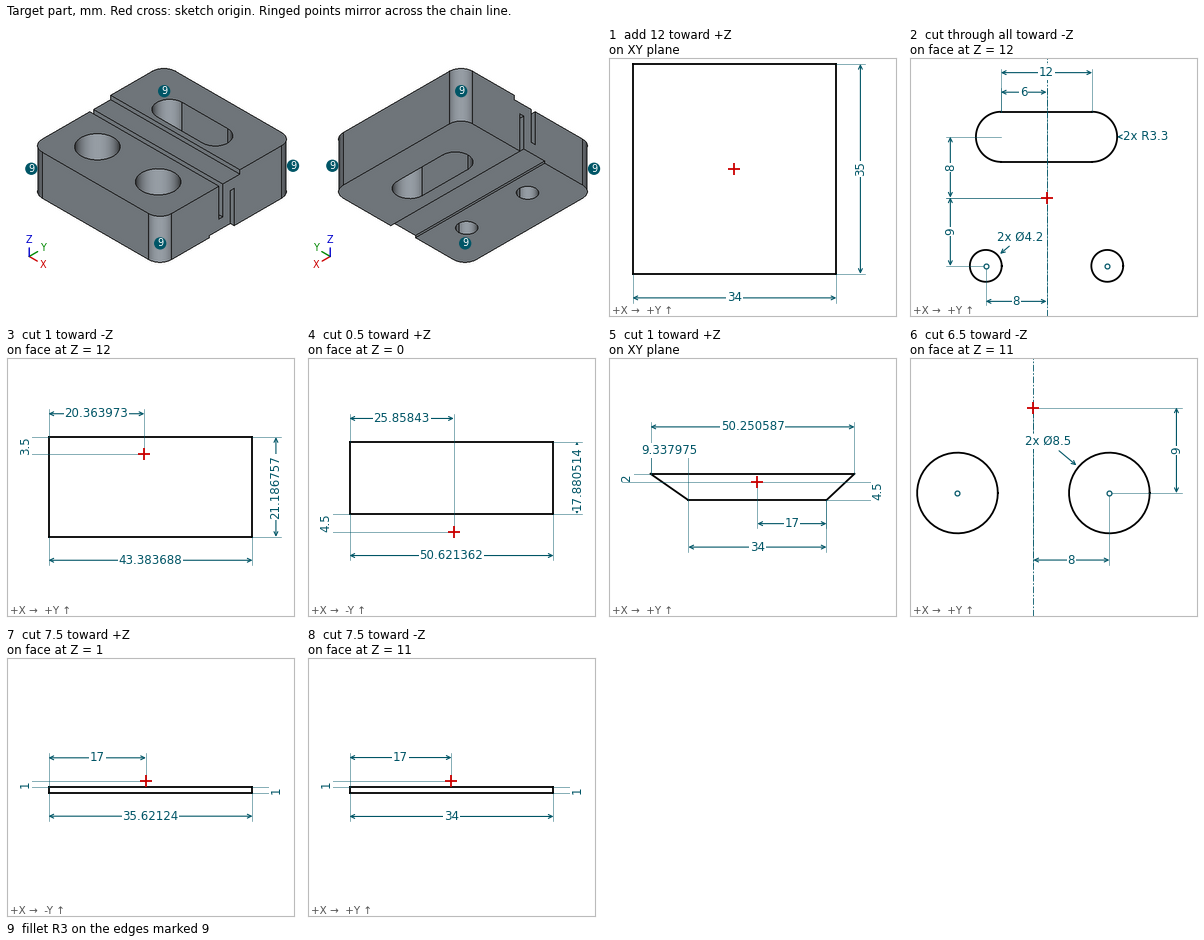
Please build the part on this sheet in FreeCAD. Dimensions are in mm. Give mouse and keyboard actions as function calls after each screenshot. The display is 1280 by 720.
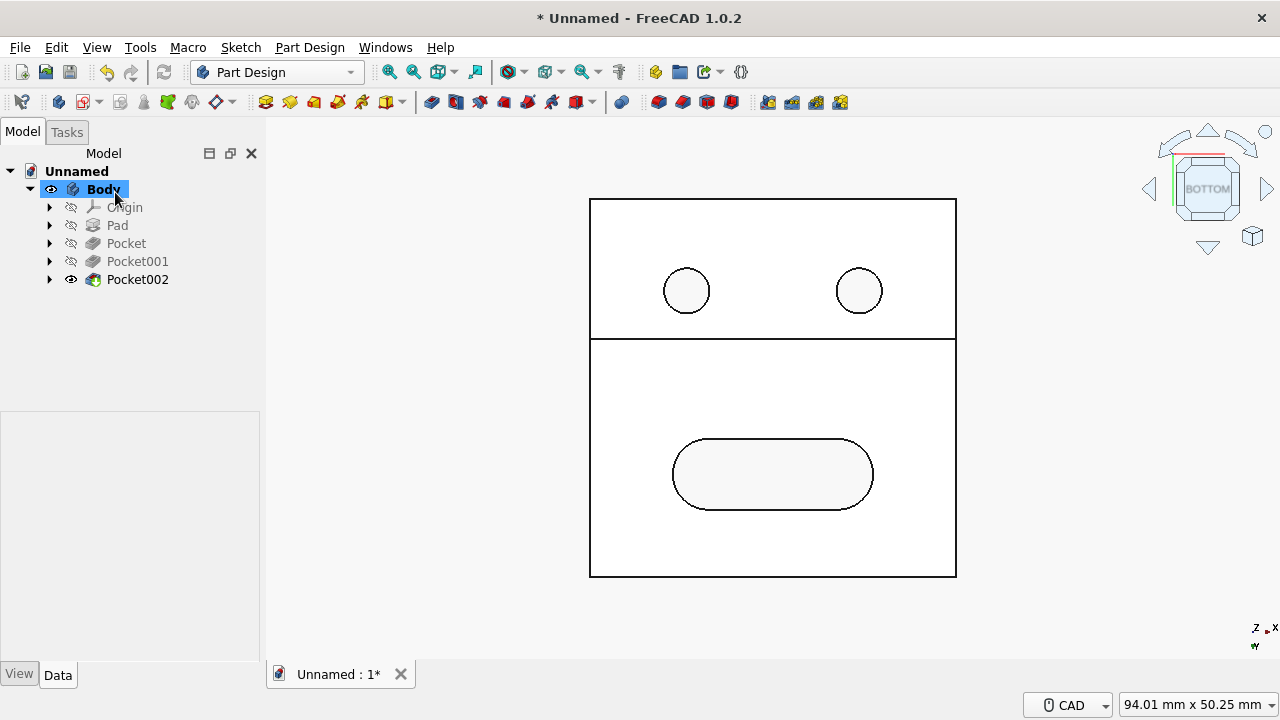
click(84, 102)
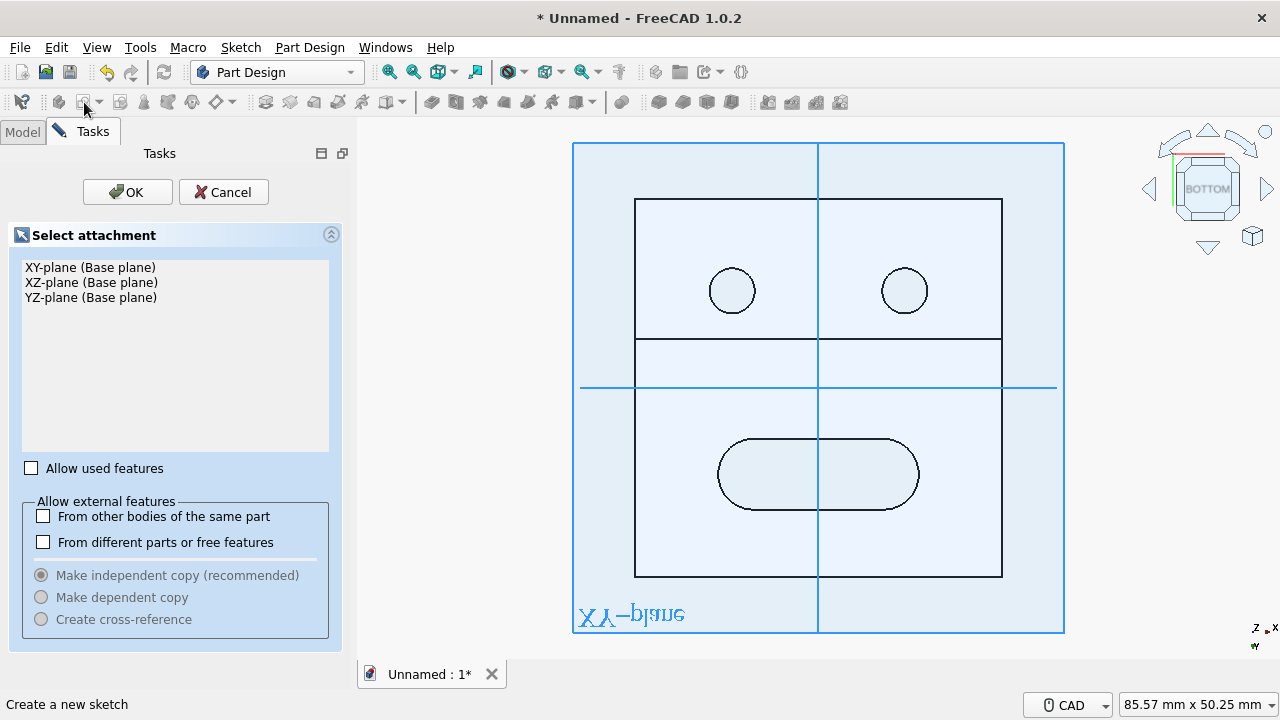
click(82, 268)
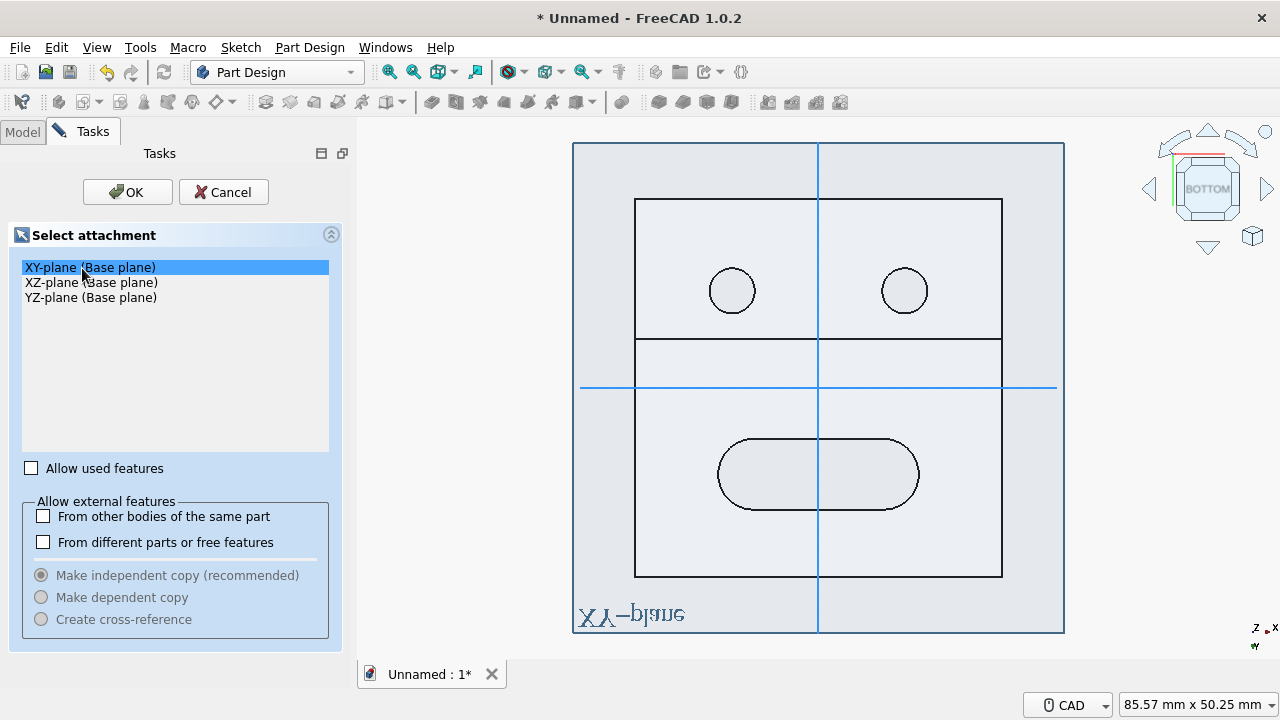
click(128, 192)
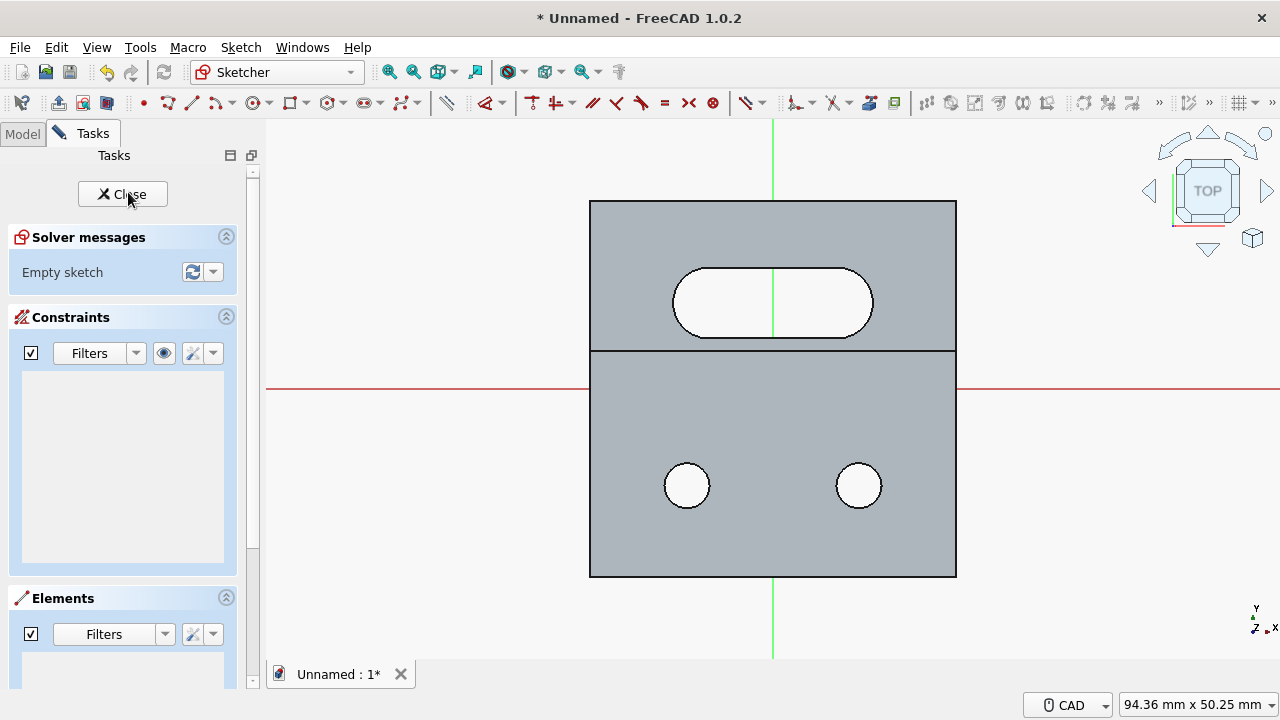
click(108, 104)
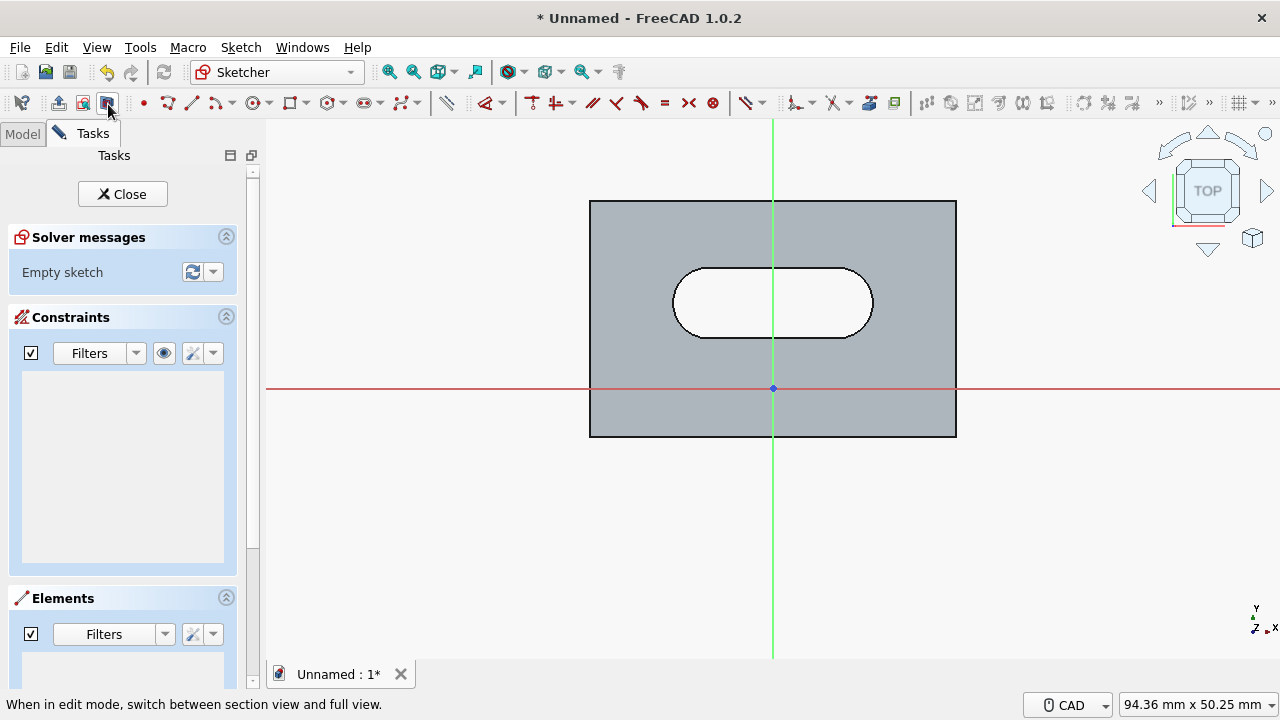
key(g)
key(m)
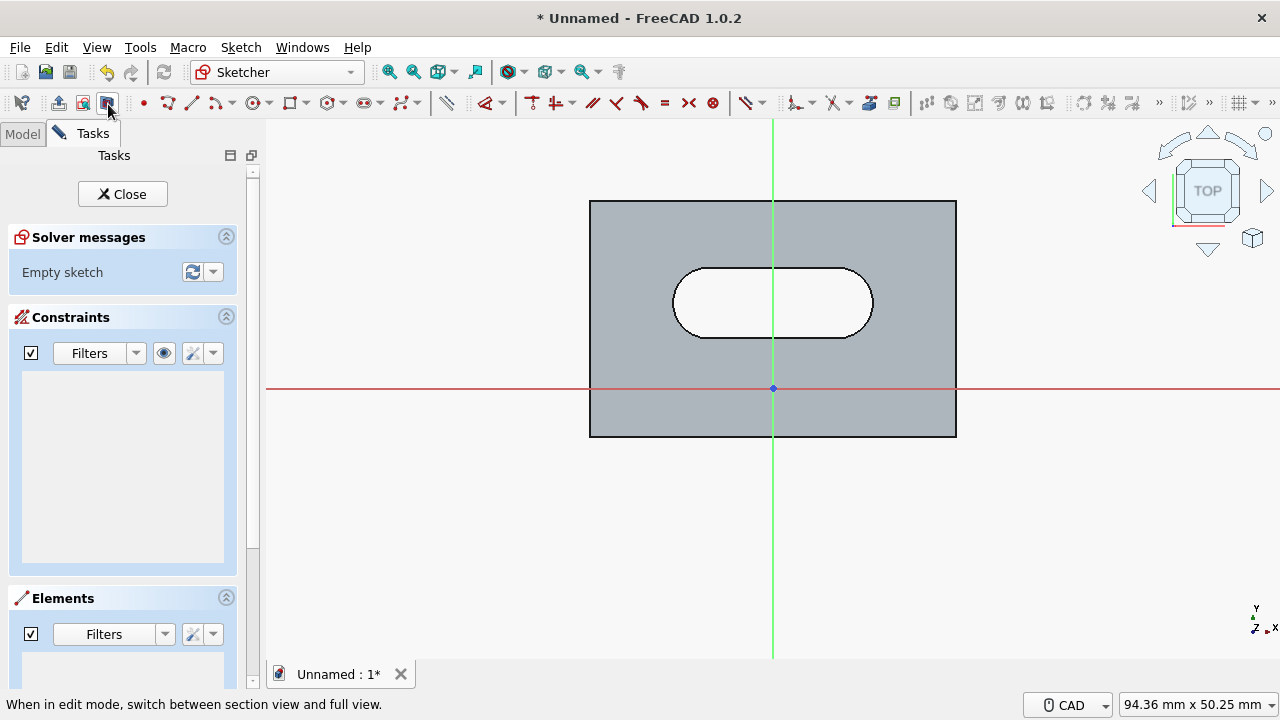
click(956, 437)
click(590, 437)
click(490, 368)
click(1030, 368)
click(956, 438)
key(Escape)
key(Escape)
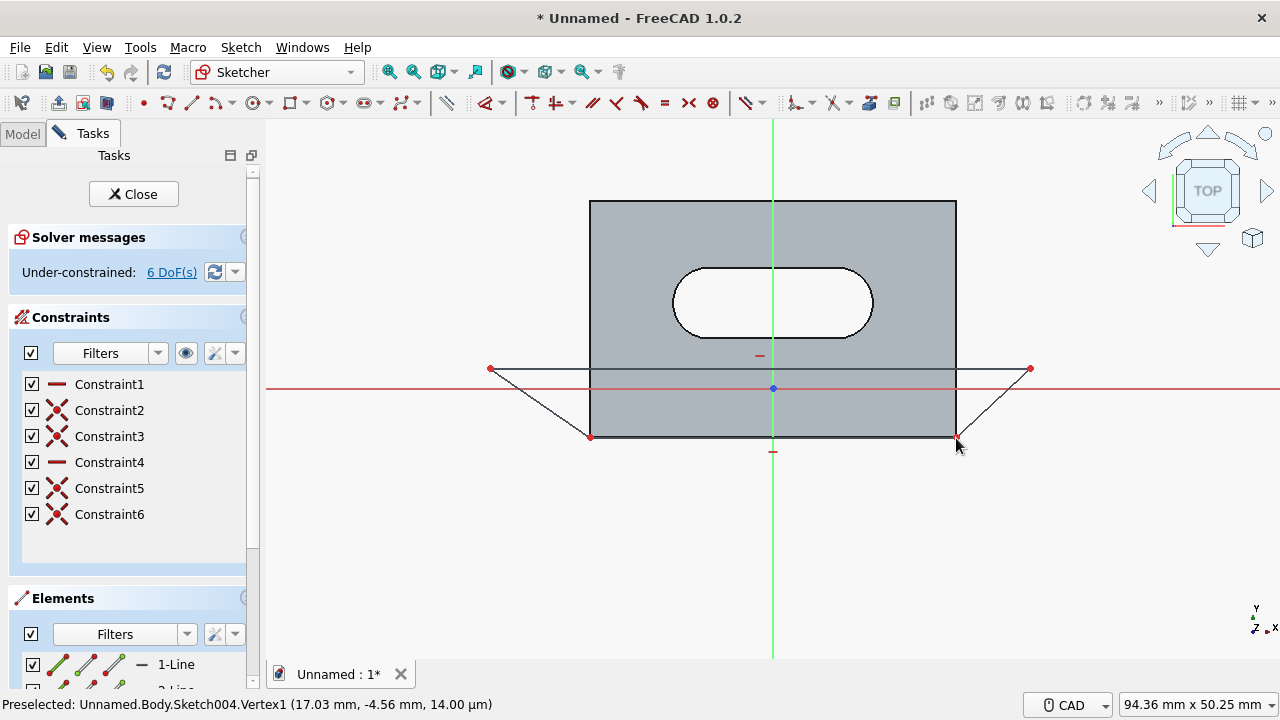
click(486, 104)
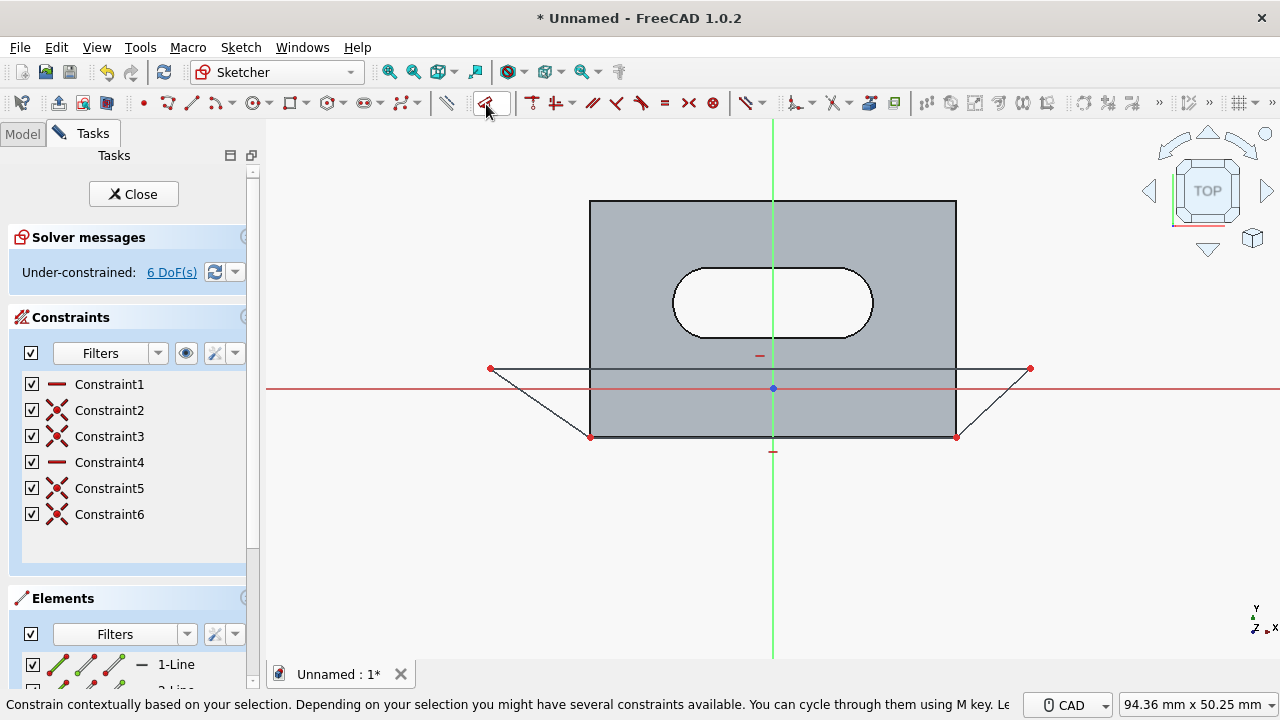
click(846, 438)
click(689, 472)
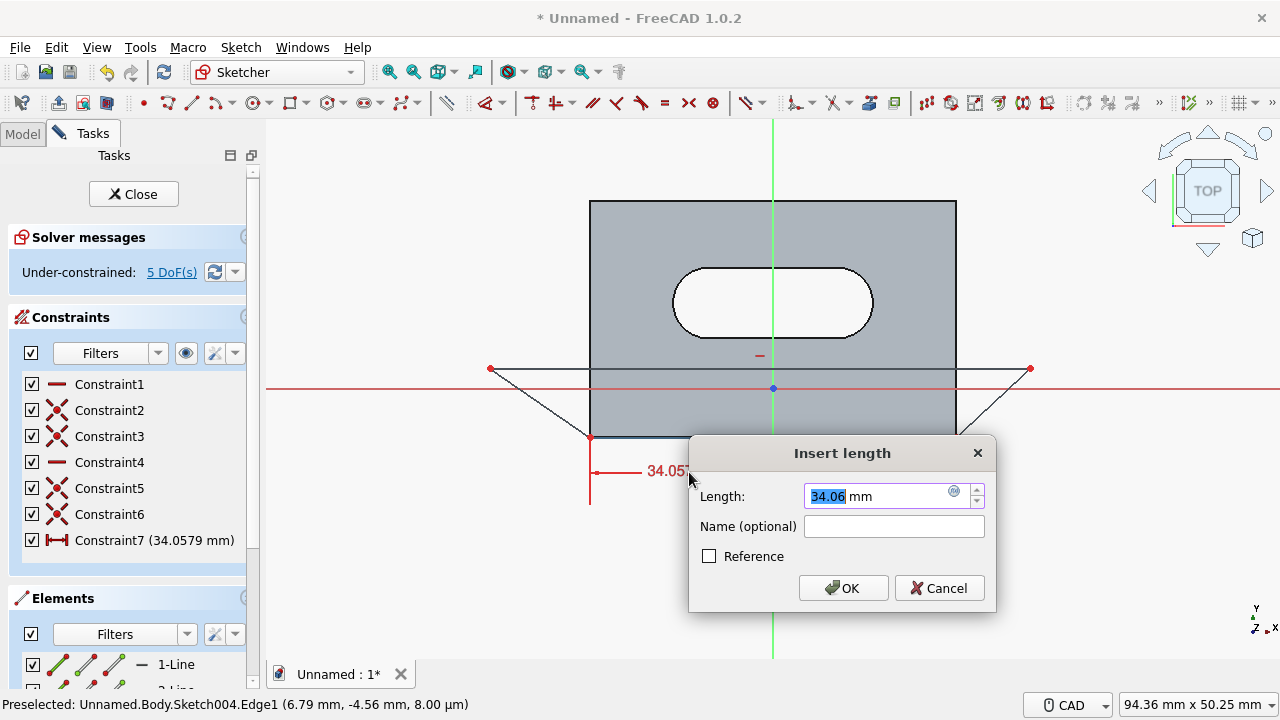
text(34)
key(Return)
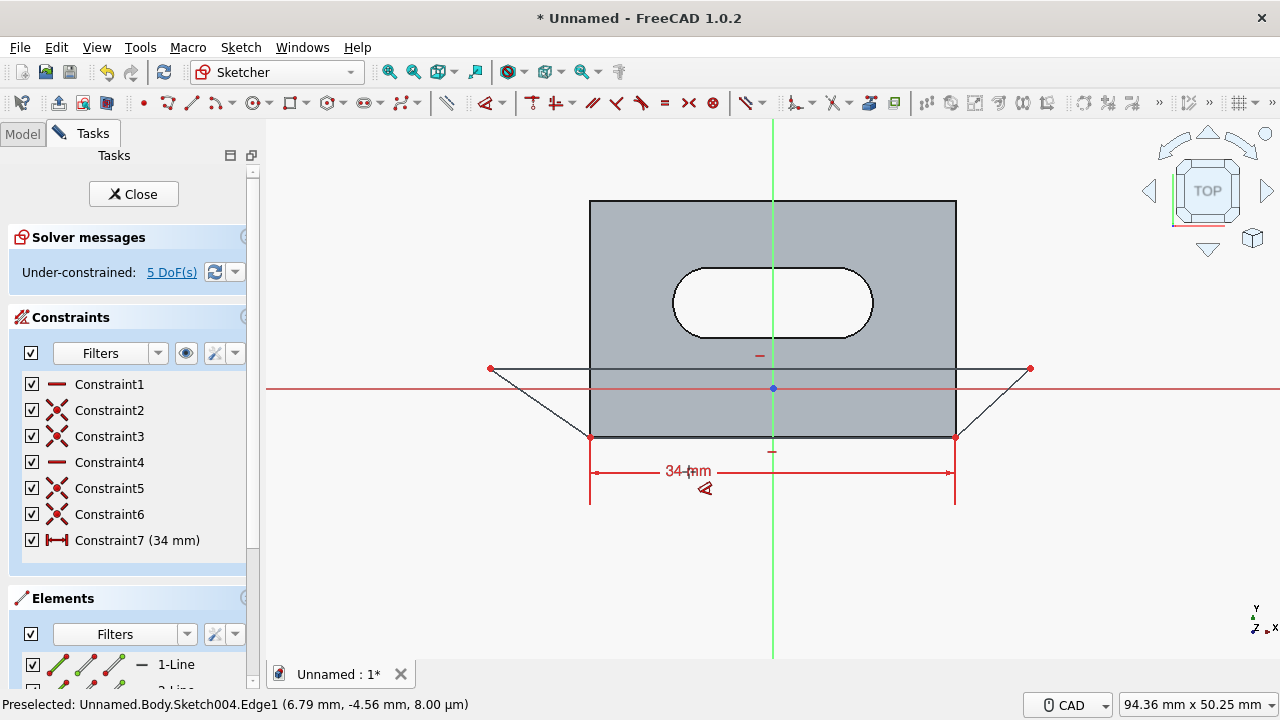
scroll(490, 369, up, 4)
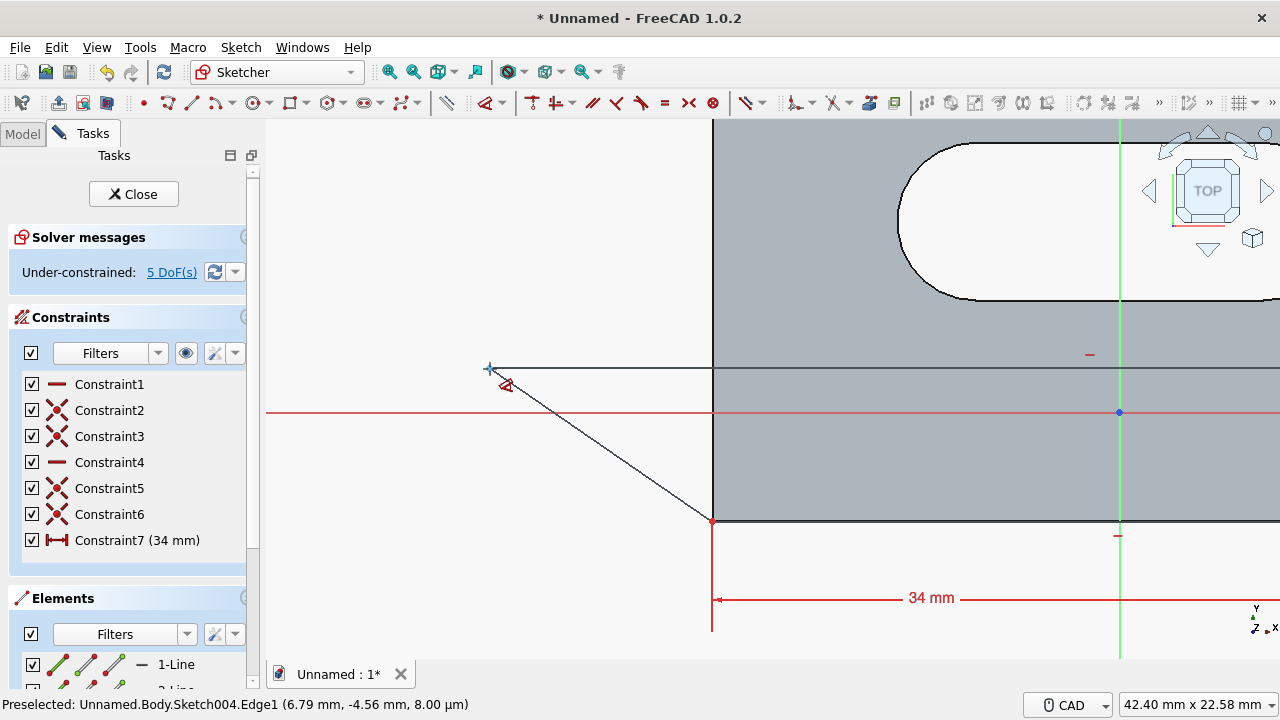
click(490, 368)
click(456, 391)